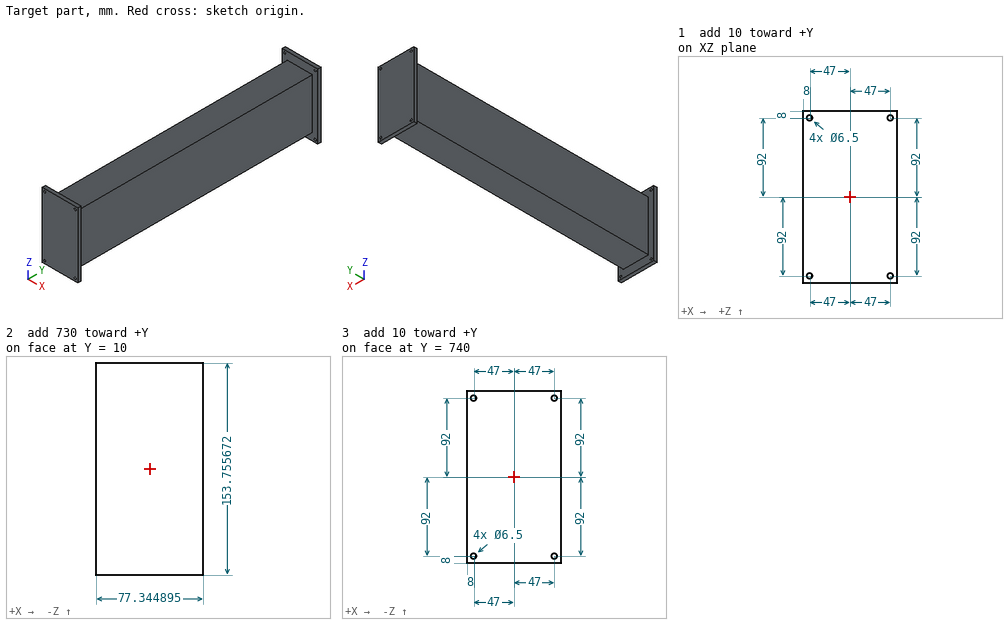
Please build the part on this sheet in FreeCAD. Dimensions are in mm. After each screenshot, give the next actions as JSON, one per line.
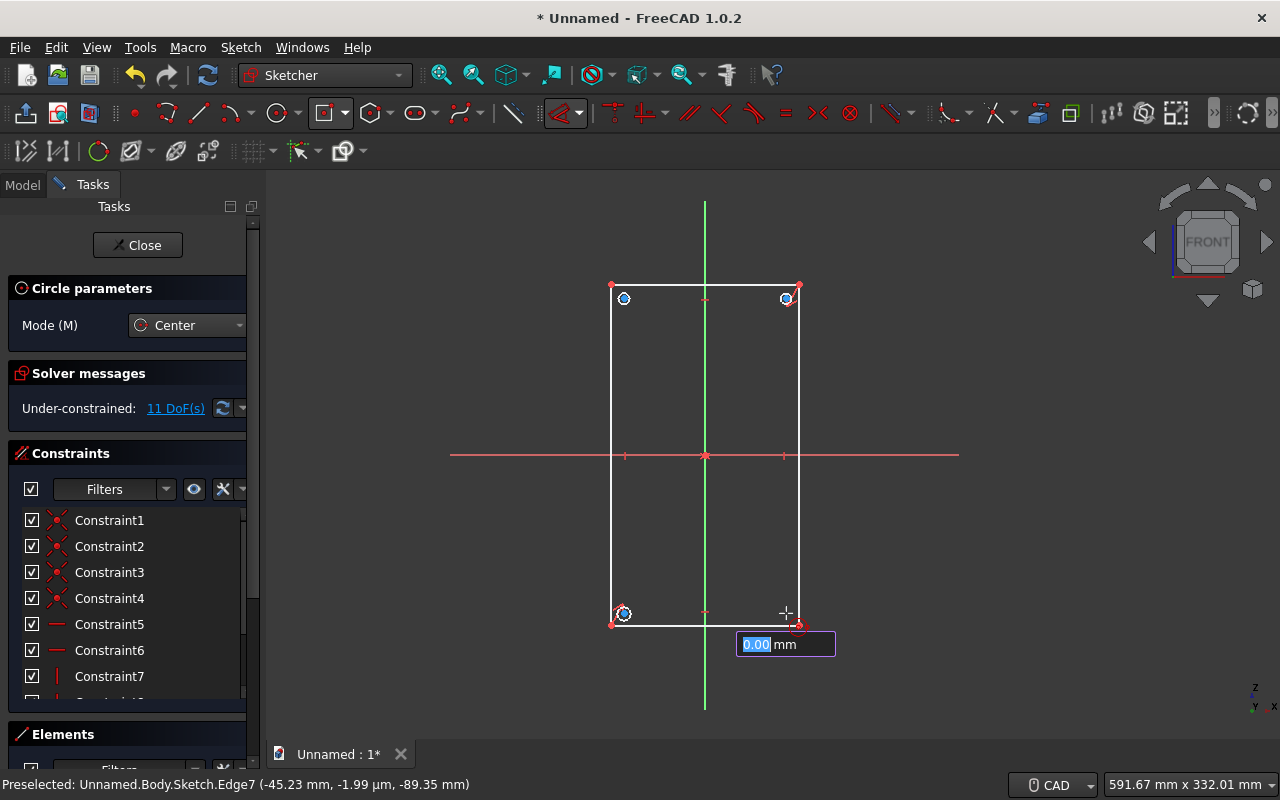
{"action": "scroll", "coordinate": [782, 609], "scroll_direction": "up", "scroll_amount": 6}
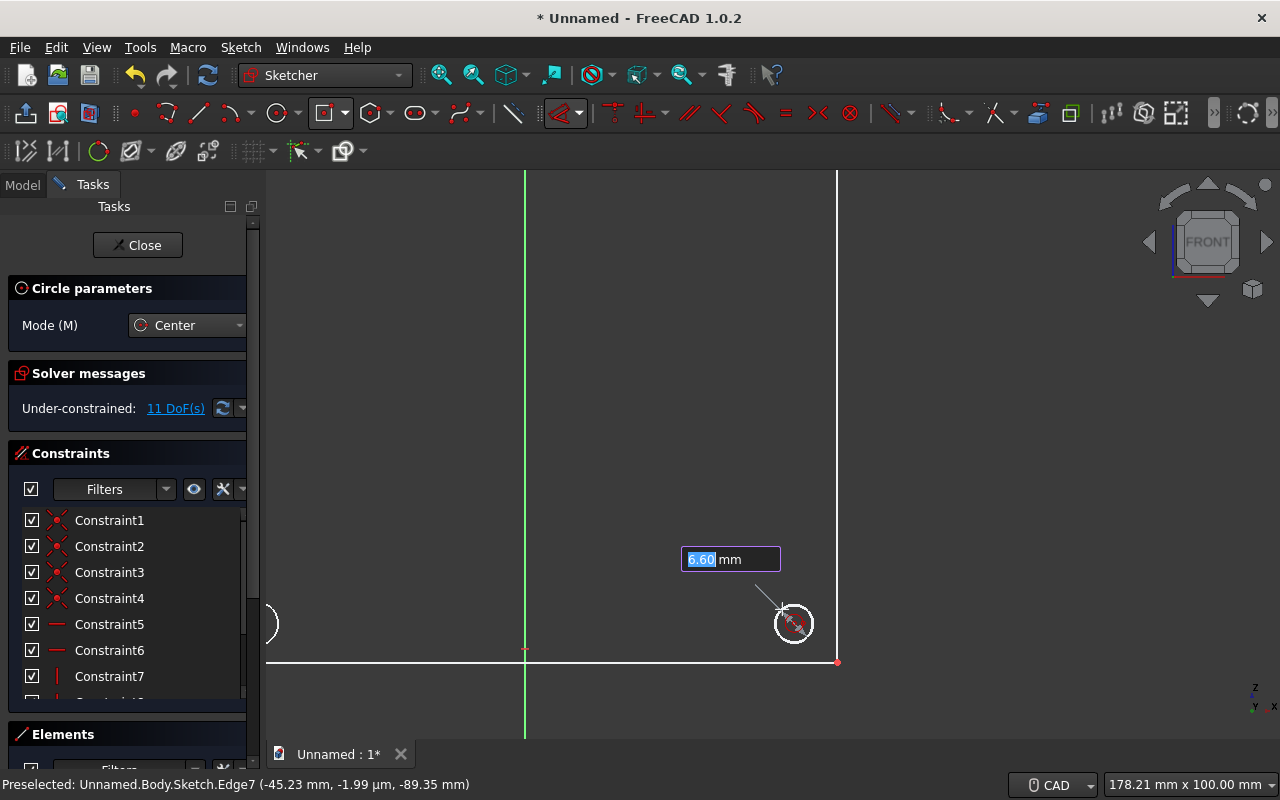
{"action": "left_click", "coordinate": [780, 607]}
{"action": "key", "text": "Escape"}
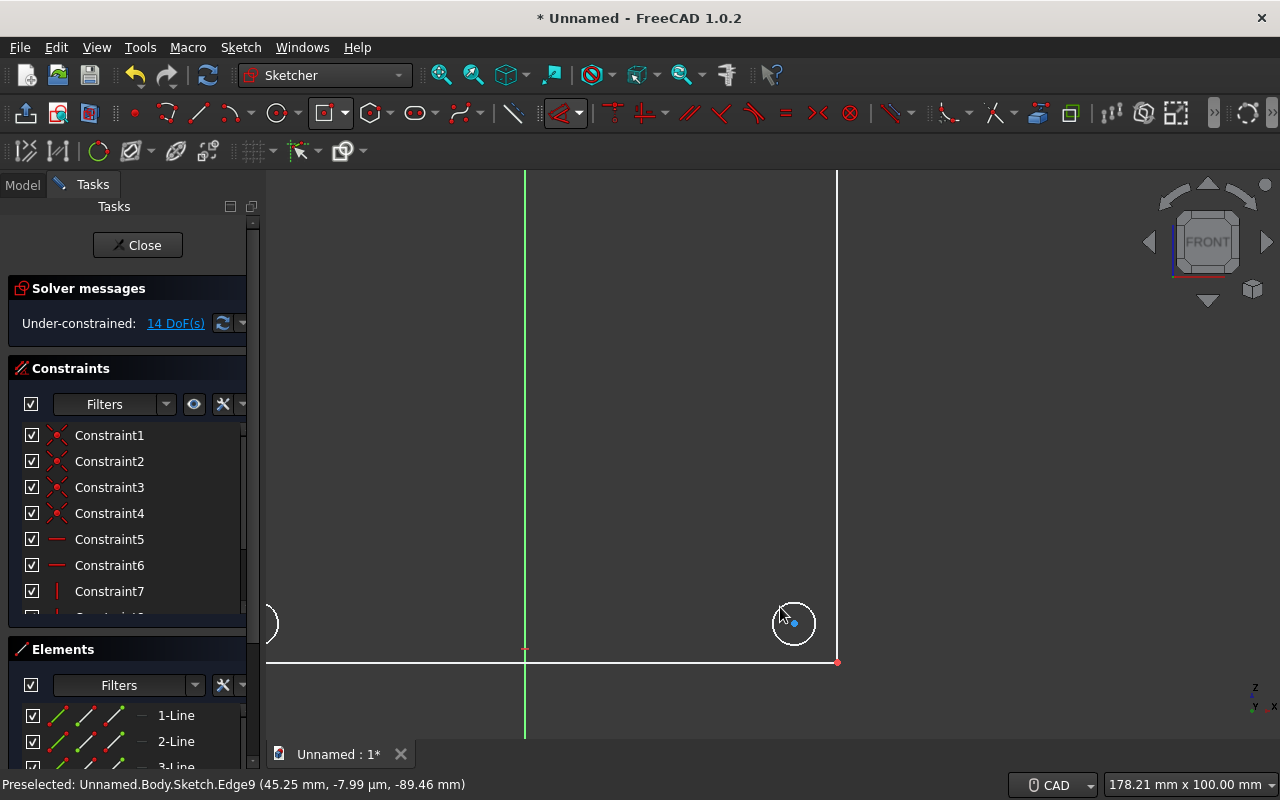
{"action": "scroll", "coordinate": [782, 609], "scroll_direction": "down", "scroll_amount": 6}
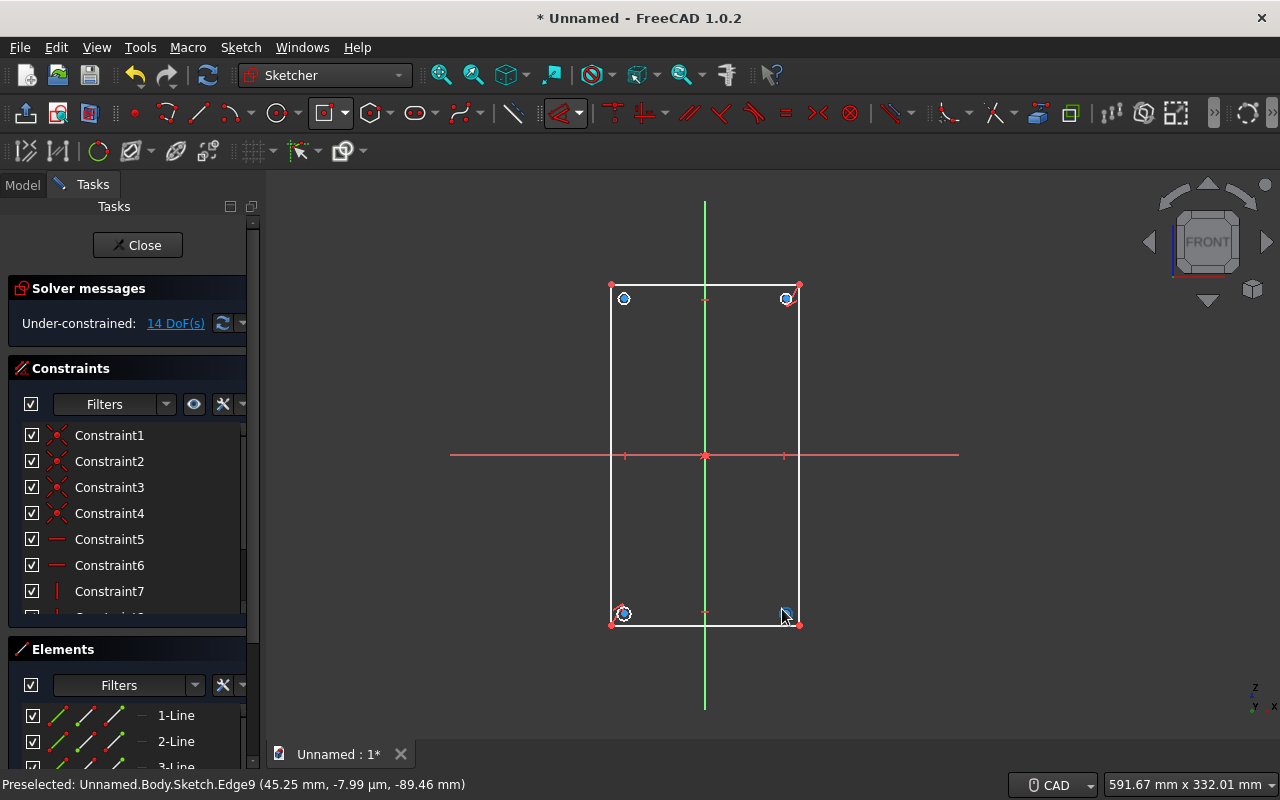
{"action": "scroll", "coordinate": [628, 295], "scroll_direction": "up", "scroll_amount": 5}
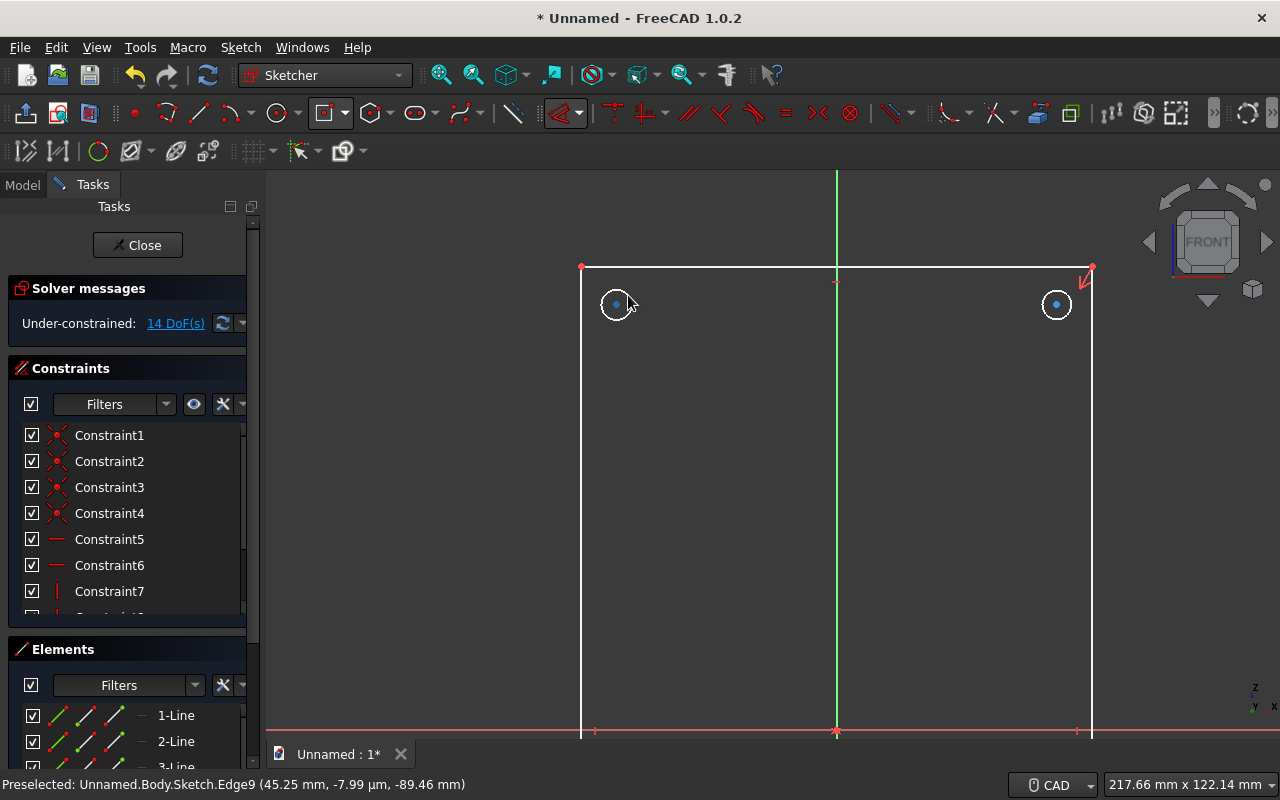
{"action": "left_click", "coordinate": [627, 294]}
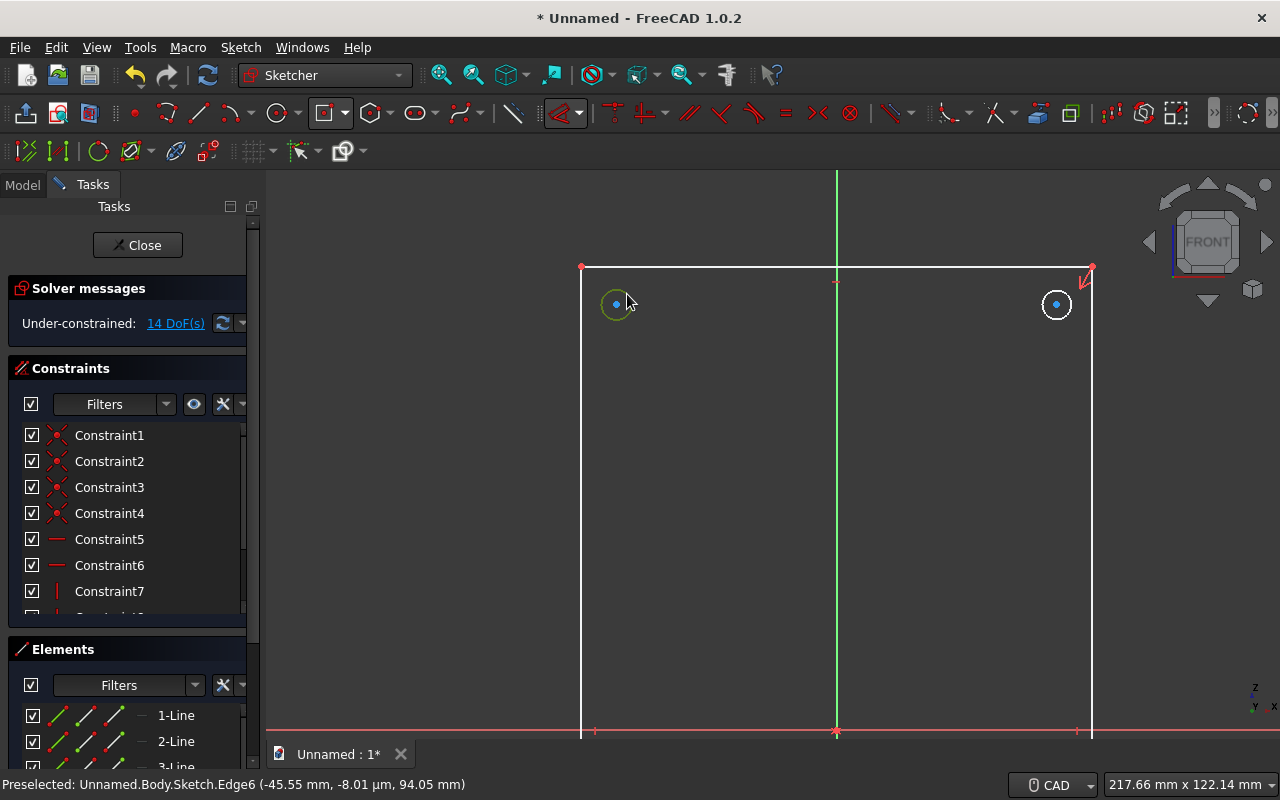
{"action": "left_click", "coordinate": [1067, 295]}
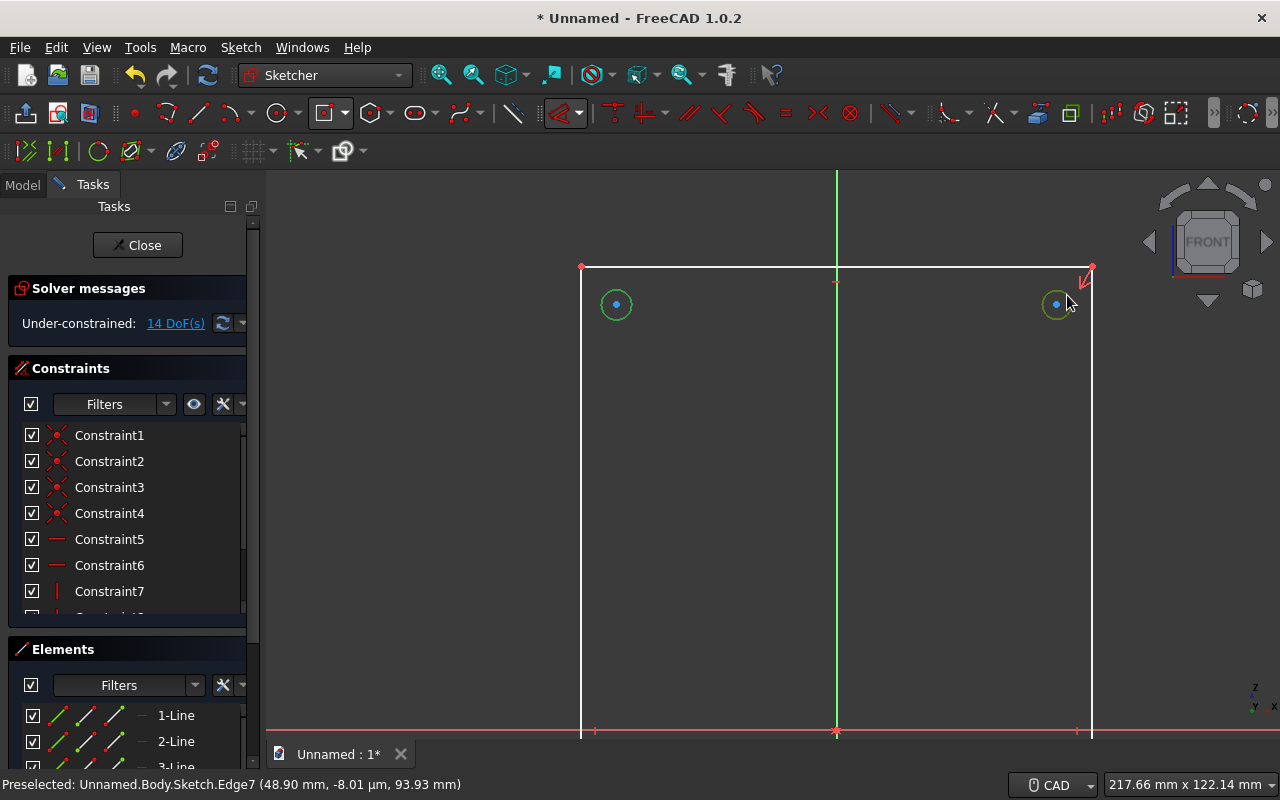
{"action": "scroll", "coordinate": [628, 294], "scroll_direction": "down", "scroll_amount": 5}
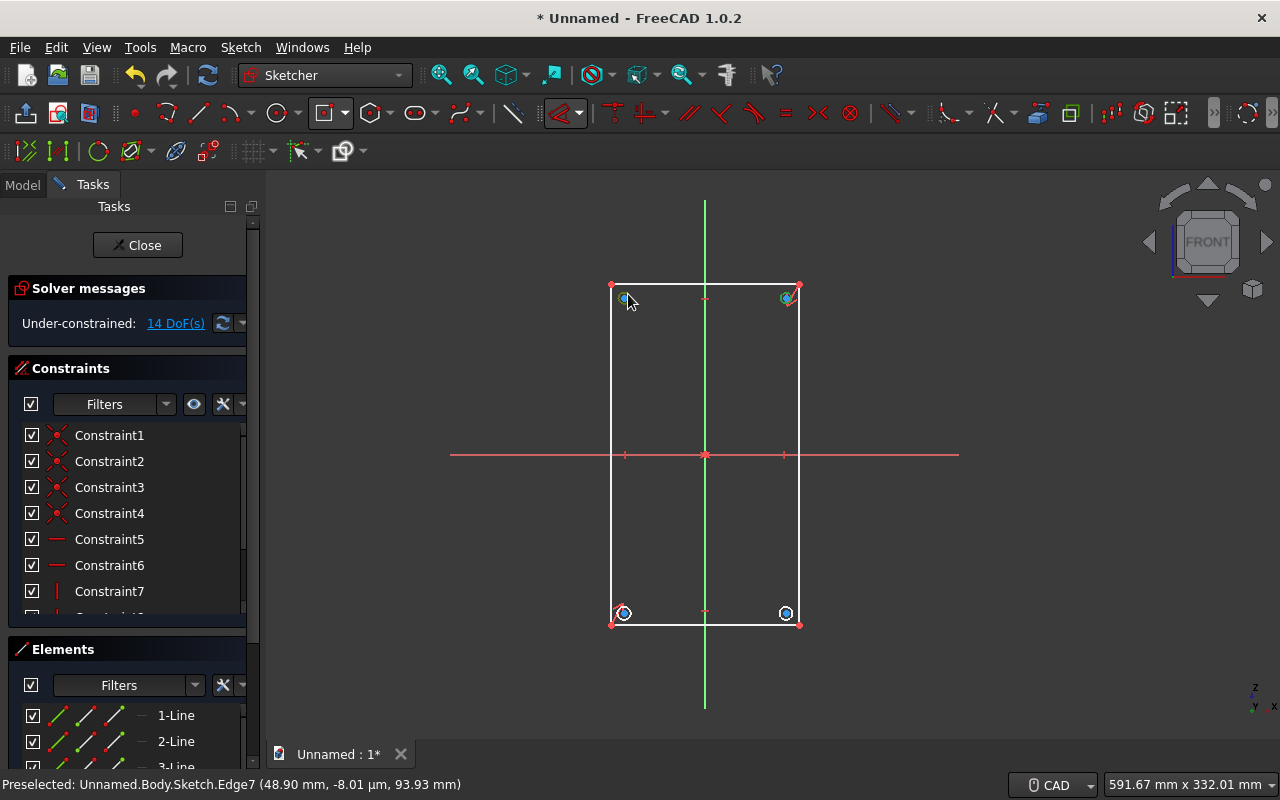
{"action": "scroll", "coordinate": [629, 609], "scroll_direction": "up", "scroll_amount": 4}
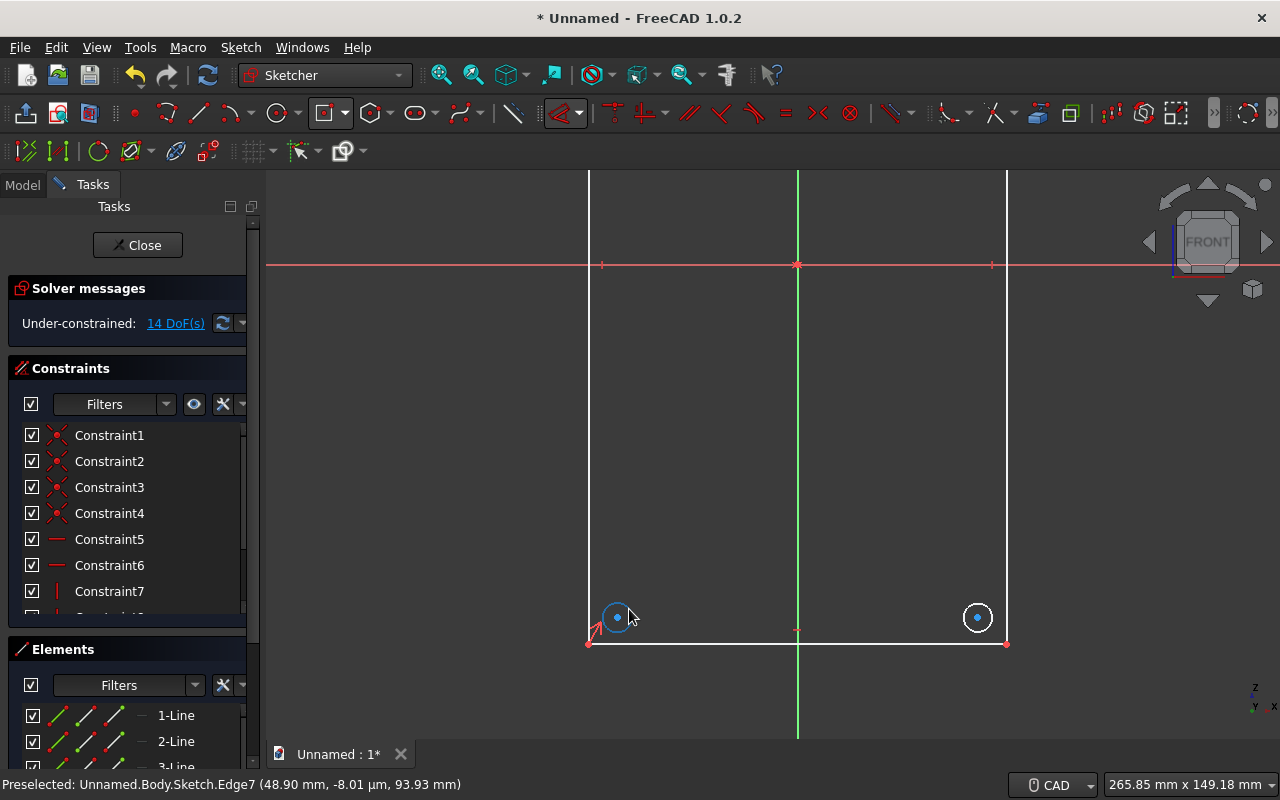
{"action": "left_click", "coordinate": [628, 607]}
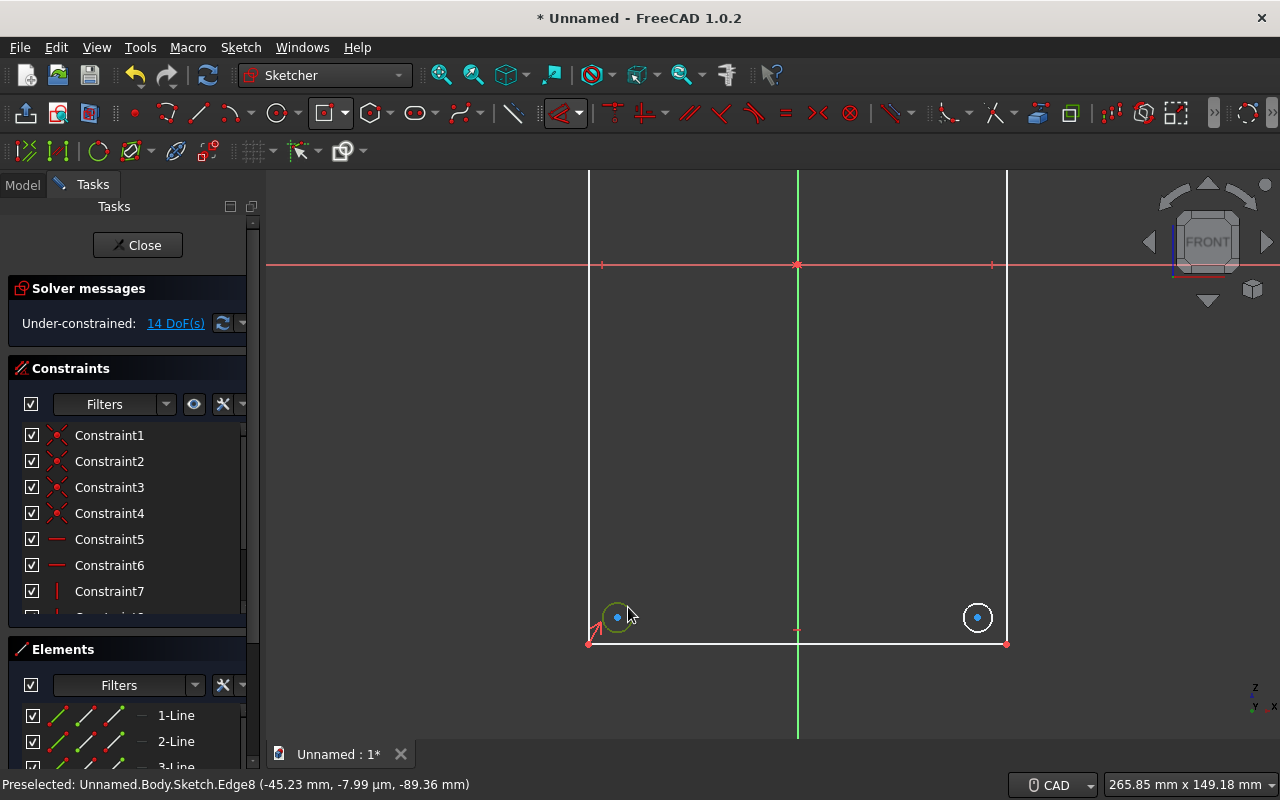
{"action": "left_click", "coordinate": [988, 608]}